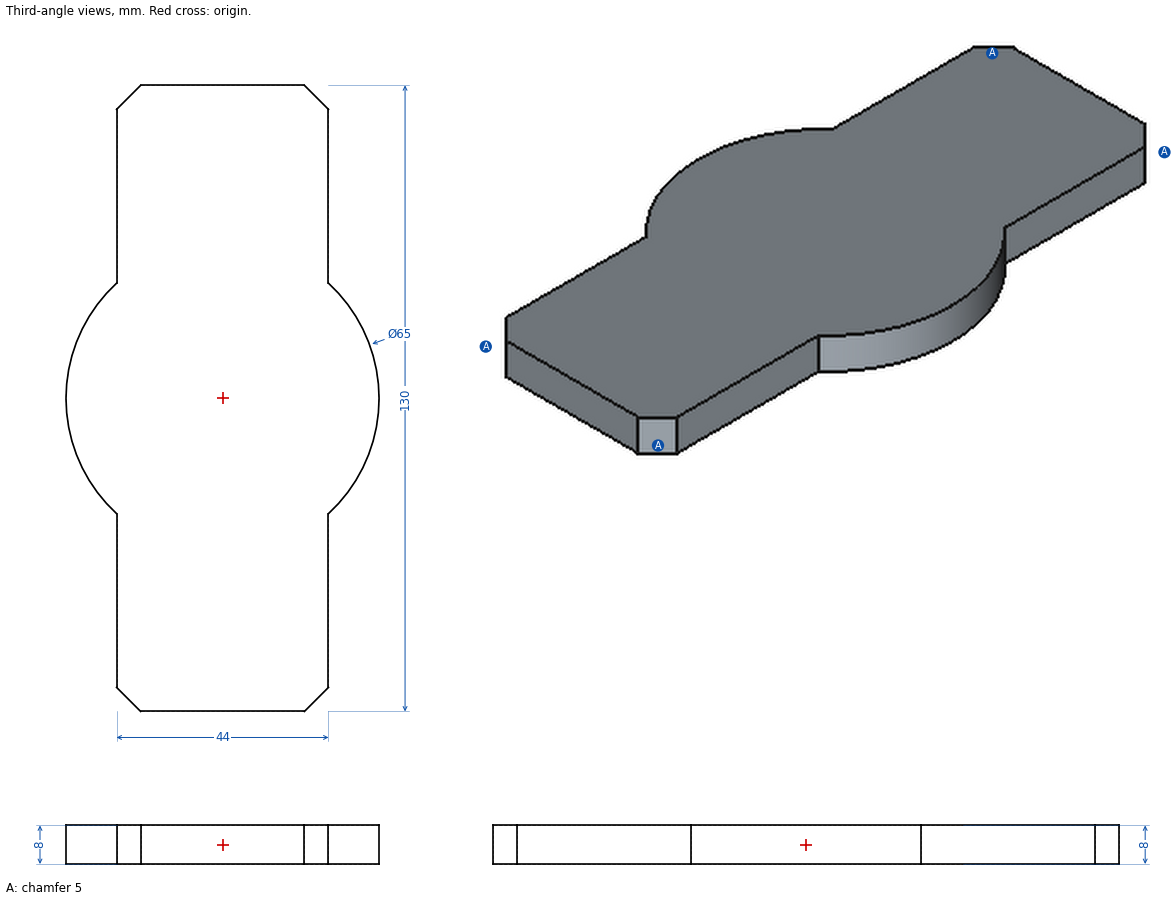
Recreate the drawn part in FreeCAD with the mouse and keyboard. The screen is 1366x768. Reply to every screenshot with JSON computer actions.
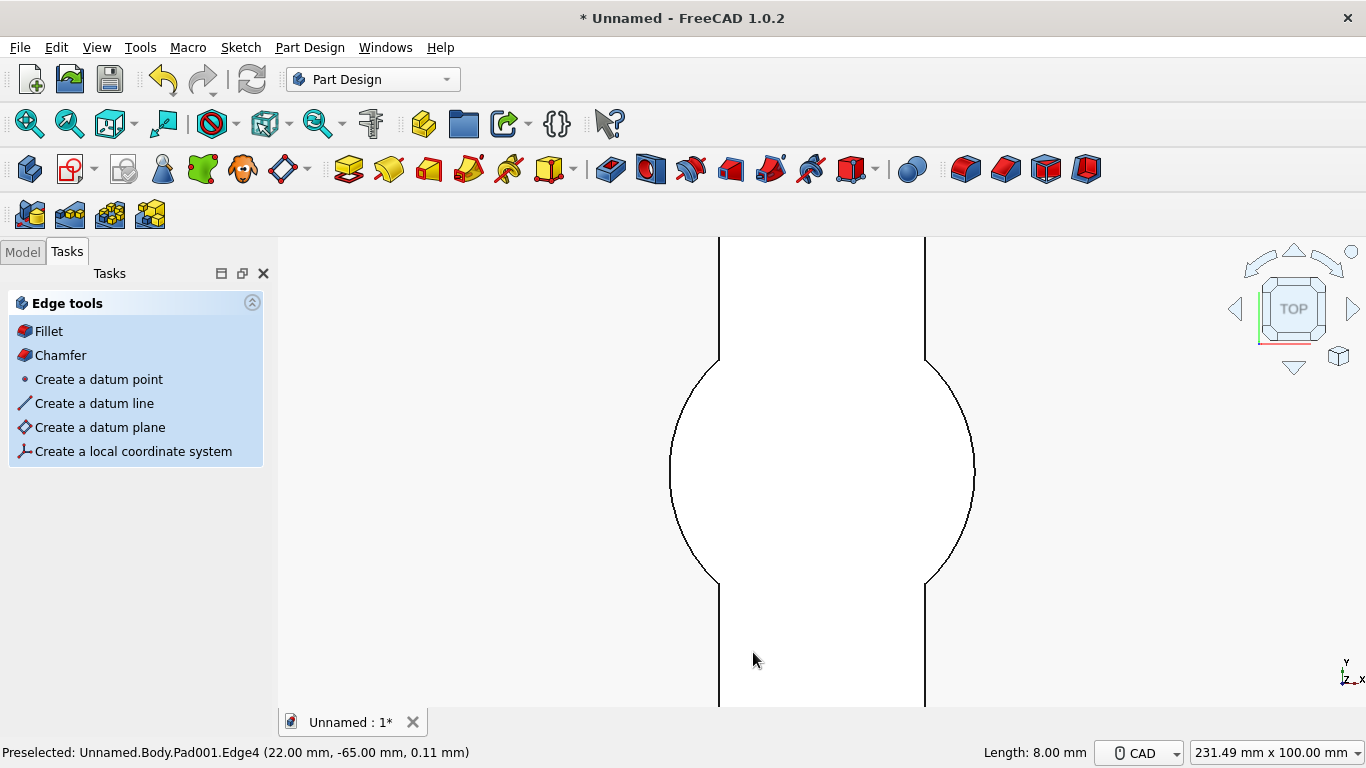
{"action": "left_click", "coordinate": [30, 124]}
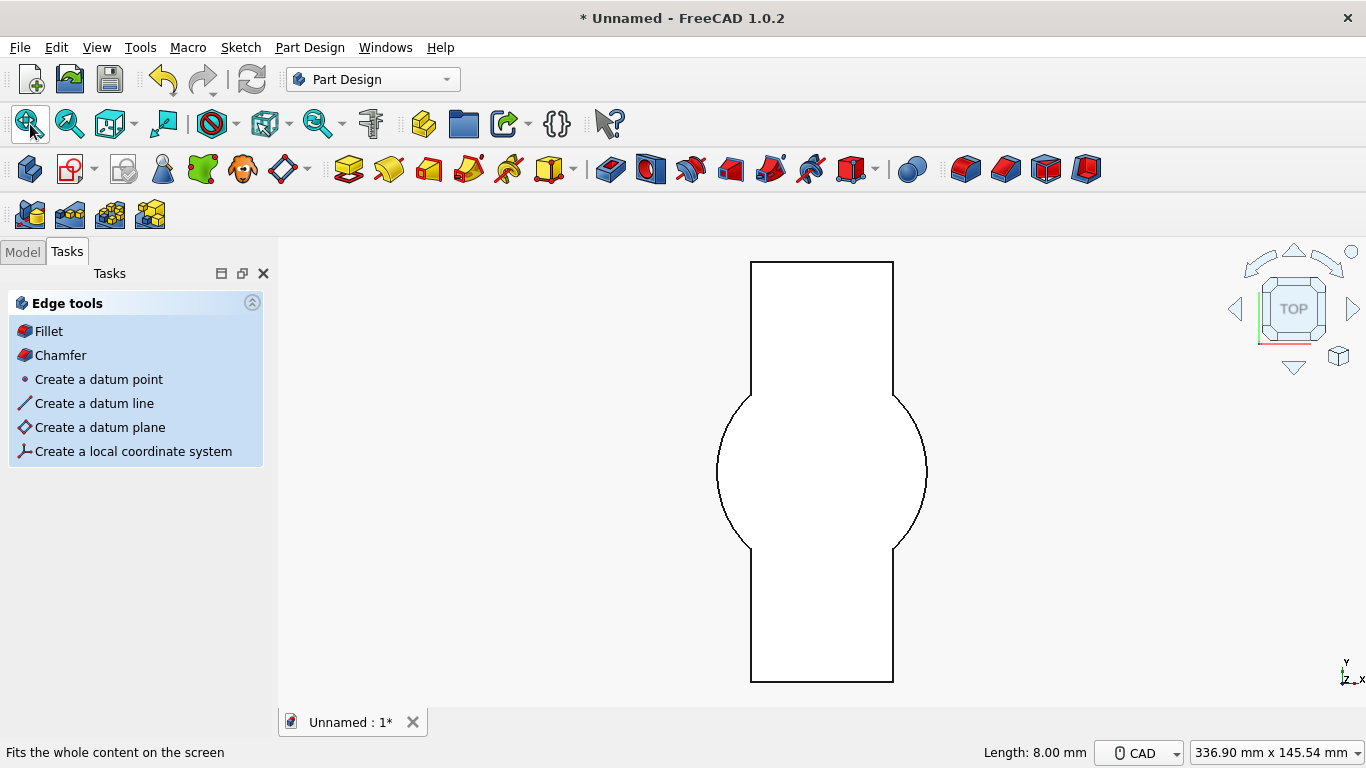
{"action": "key", "text": "1"}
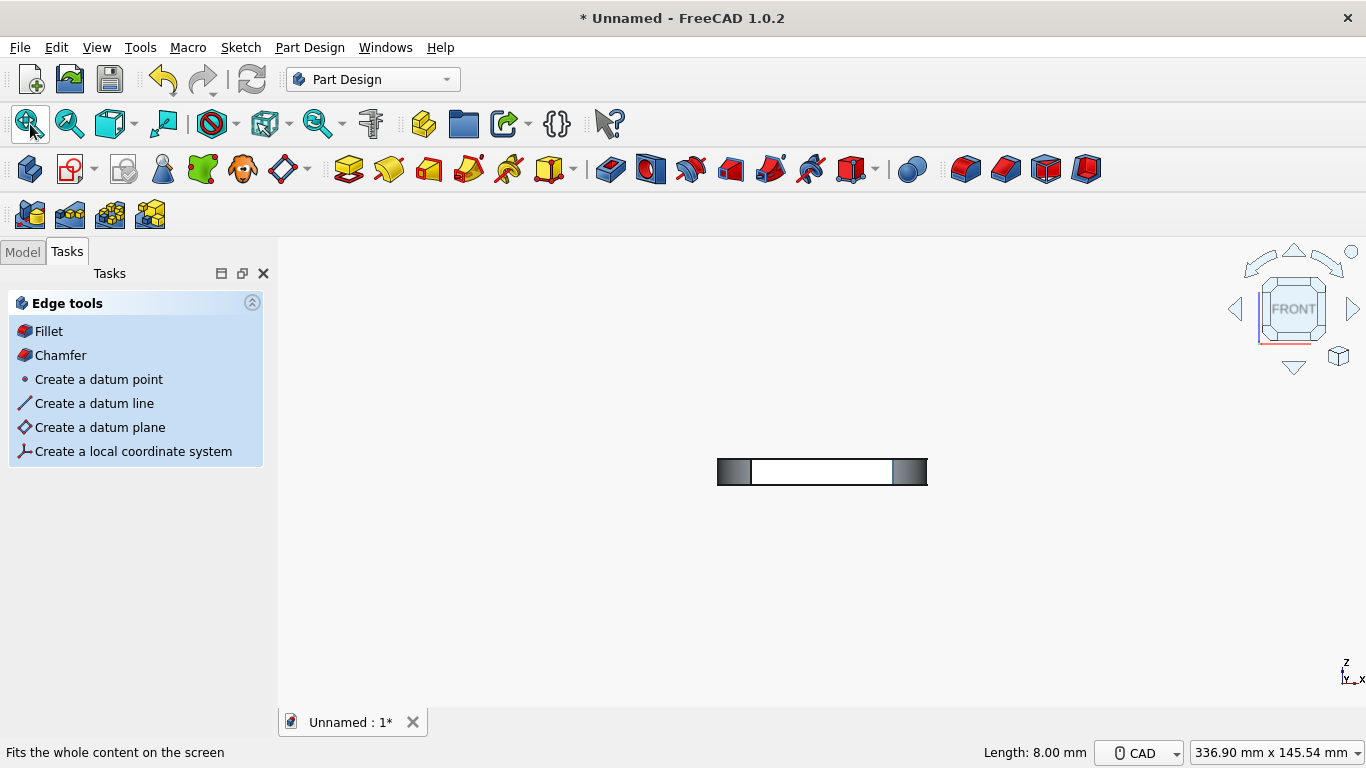
{"action": "left_click", "coordinate": [30, 124]}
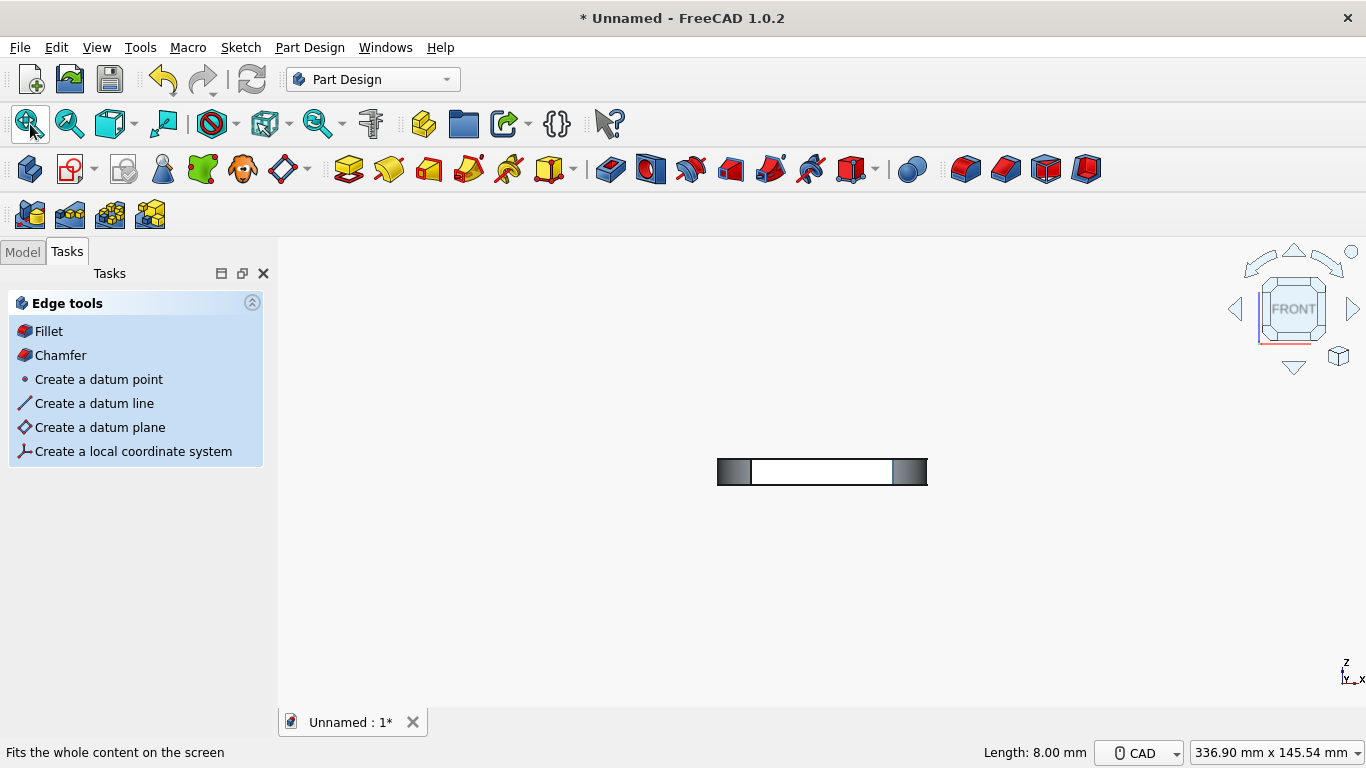
{"action": "left_click", "coordinate": [751, 471], "text": "ctrl"}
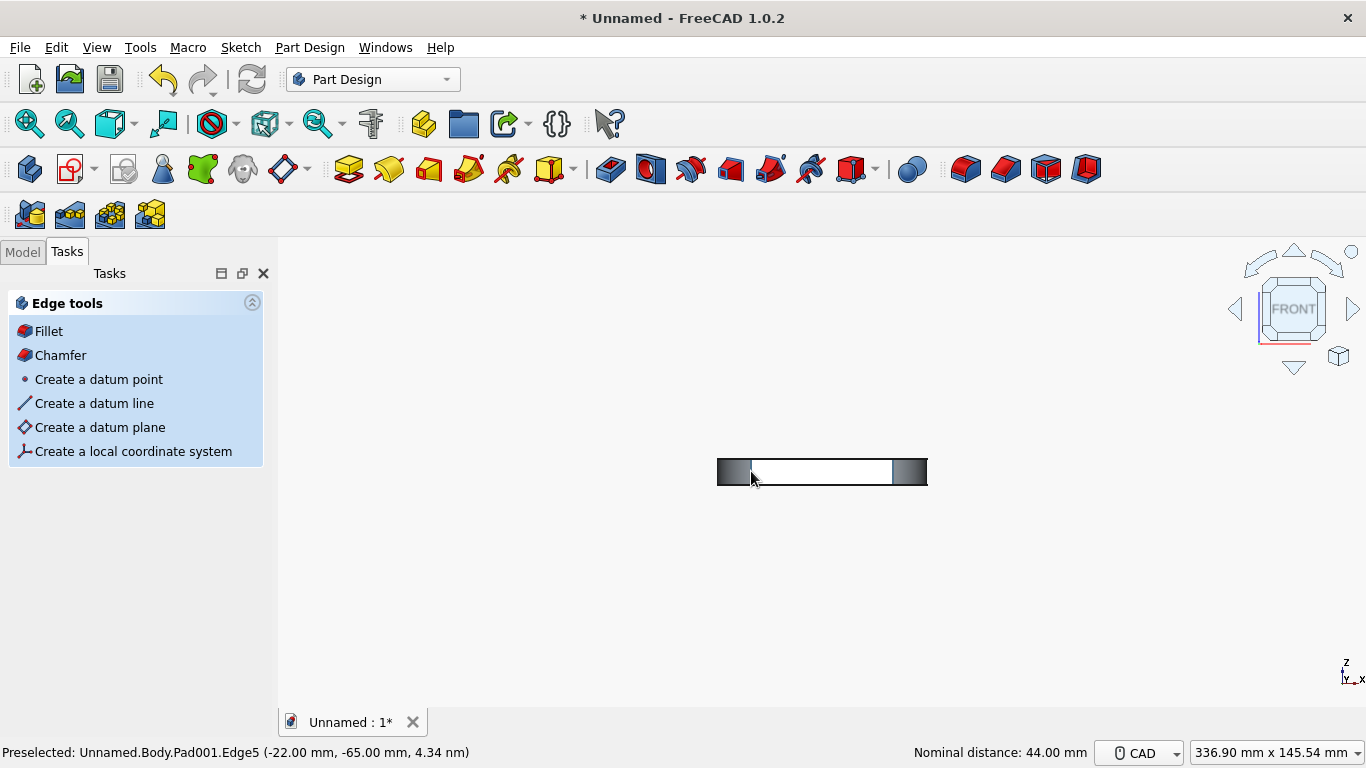
{"action": "key", "text": "3"}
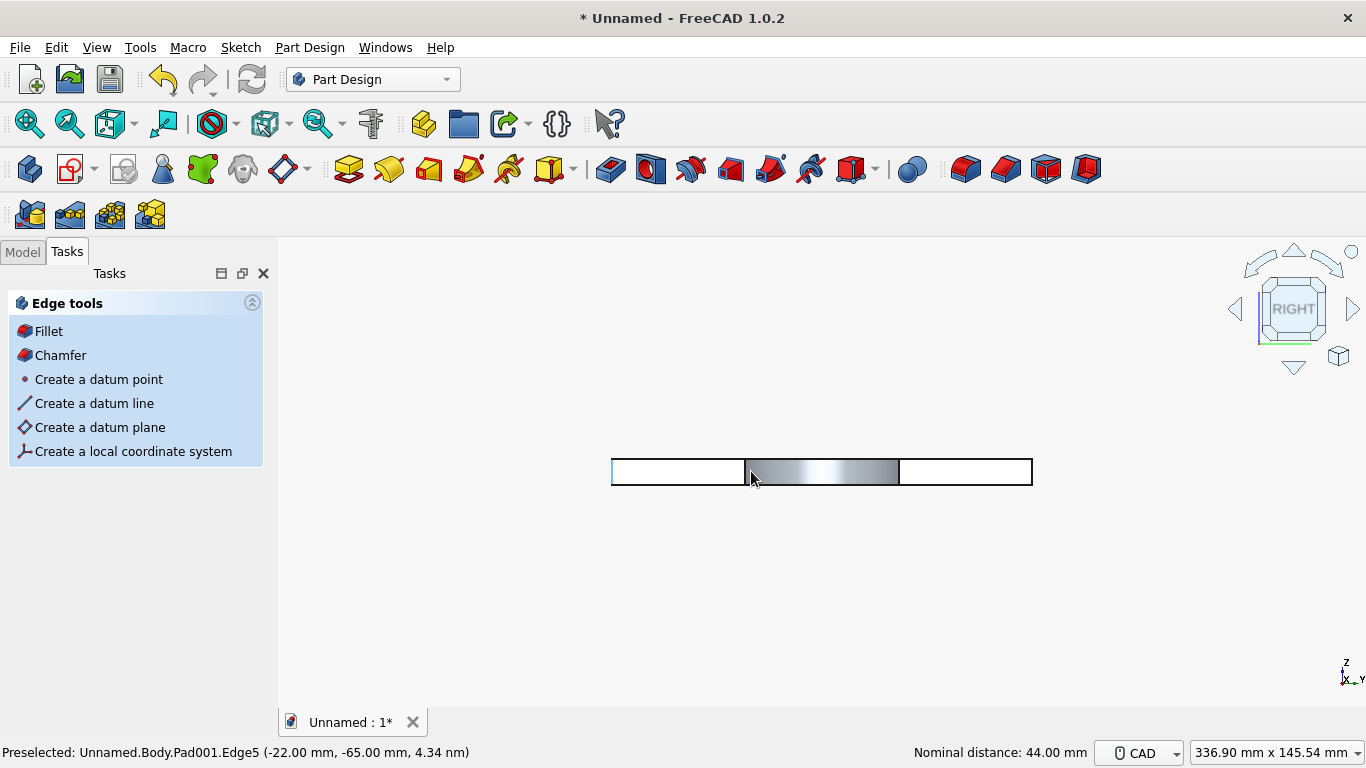
{"action": "left_click", "coordinate": [30, 124]}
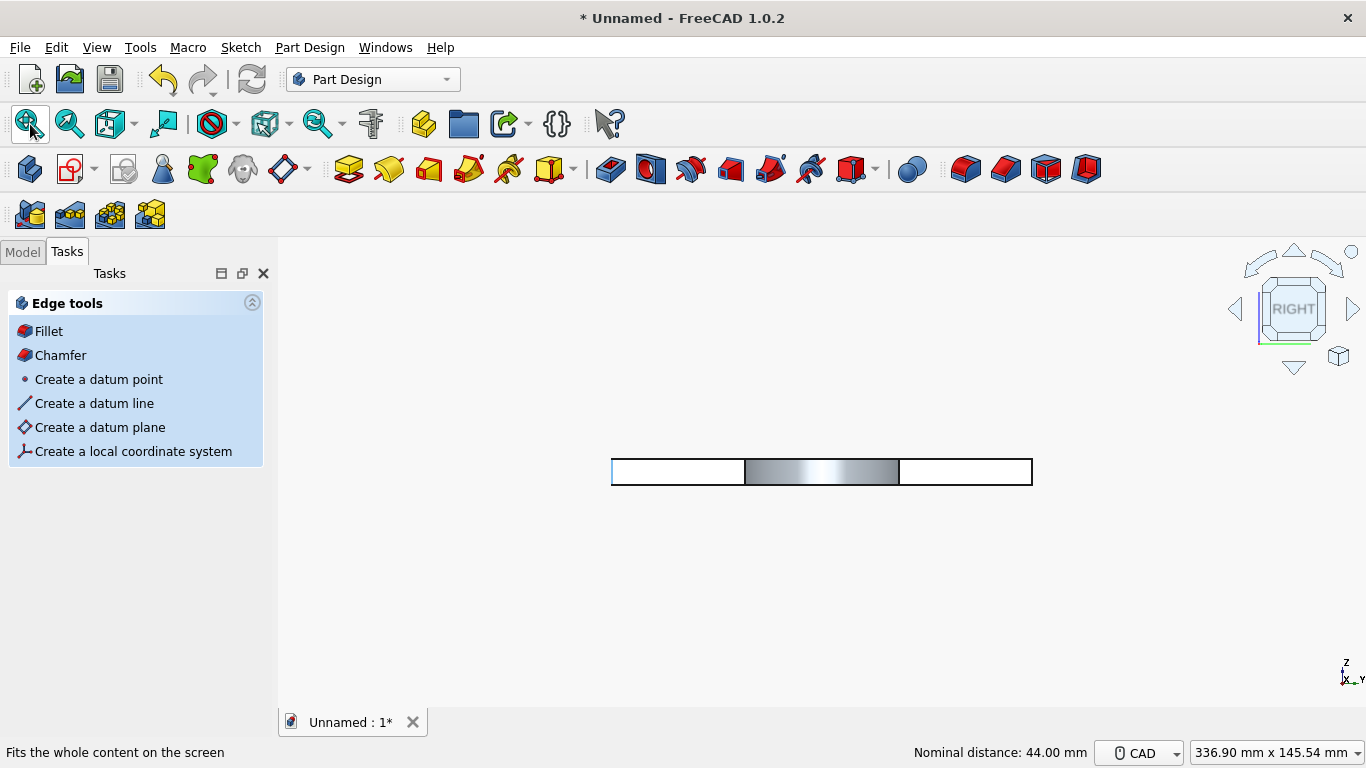
{"action": "left_click", "coordinate": [1032, 471], "text": "ctrl"}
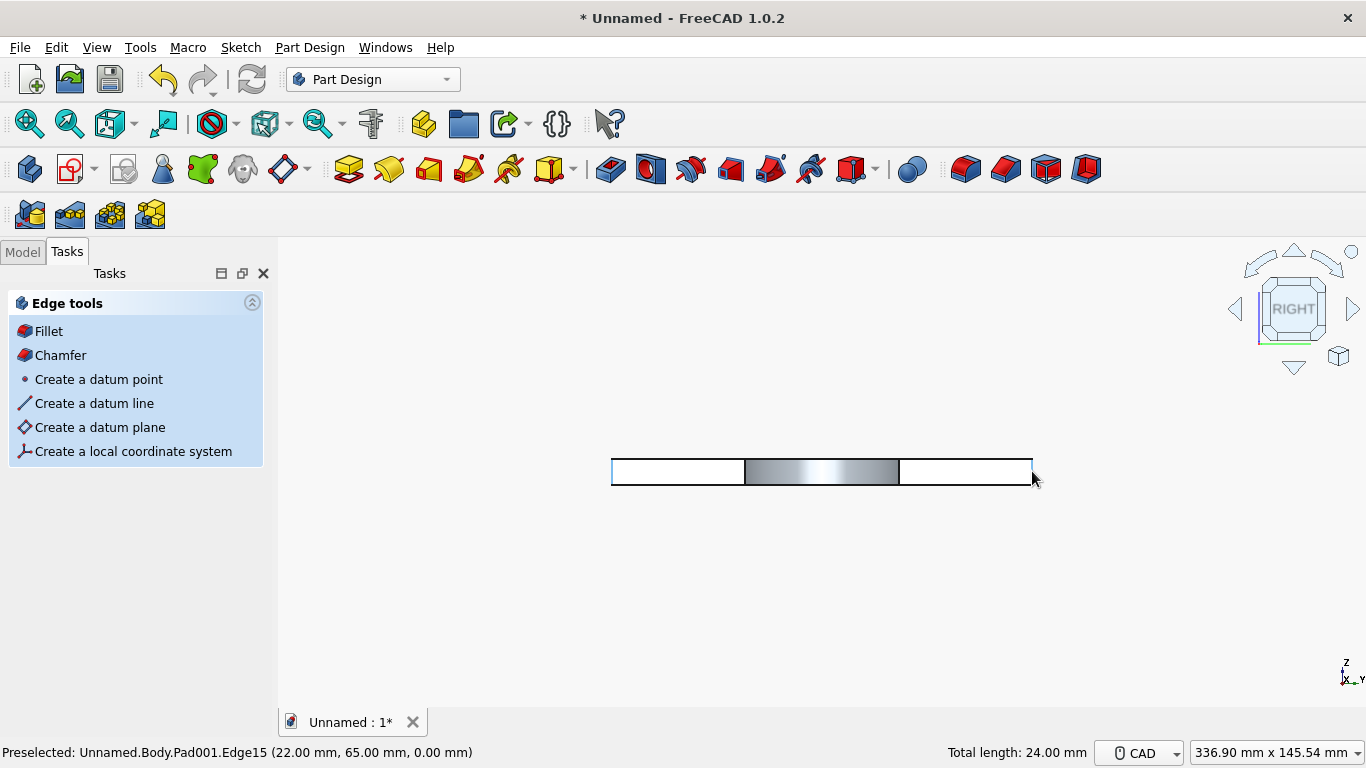
{"action": "key", "text": "5"}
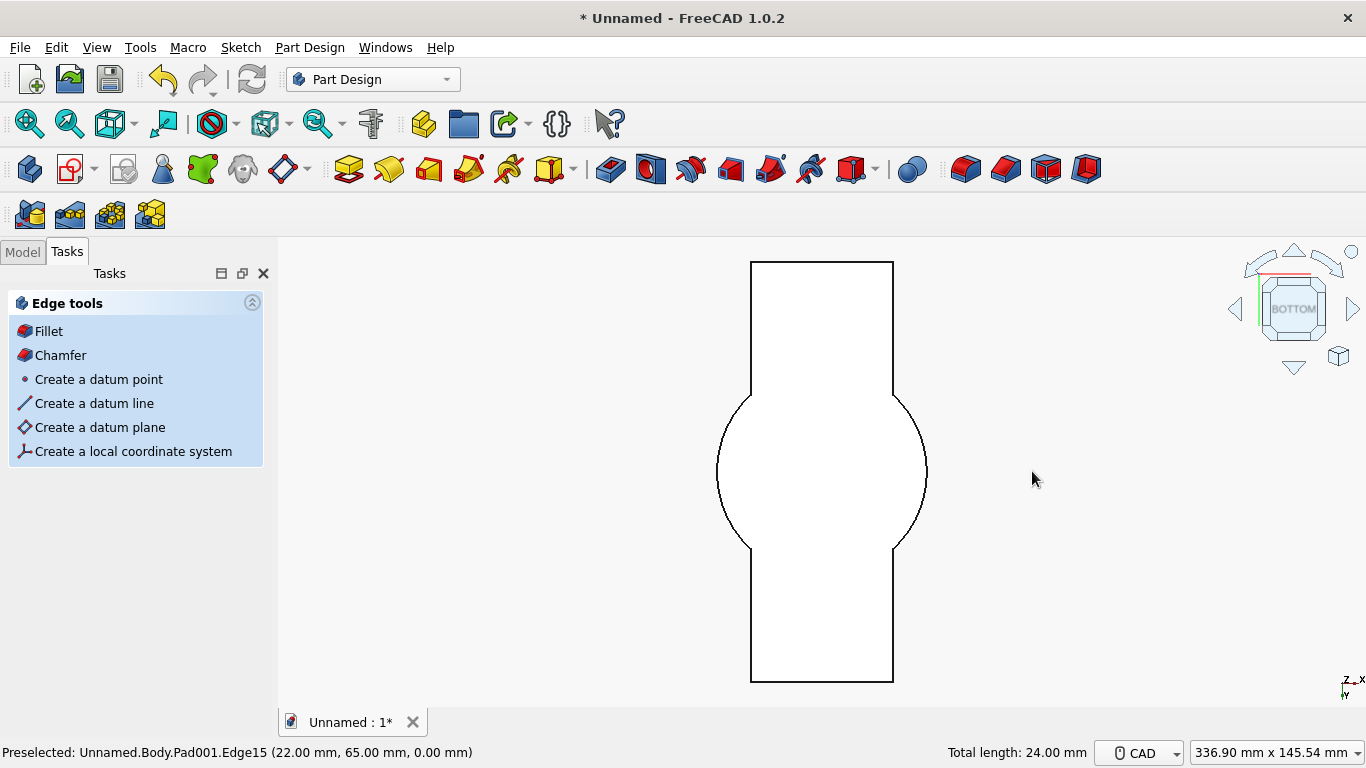
{"action": "key", "text": "4"}